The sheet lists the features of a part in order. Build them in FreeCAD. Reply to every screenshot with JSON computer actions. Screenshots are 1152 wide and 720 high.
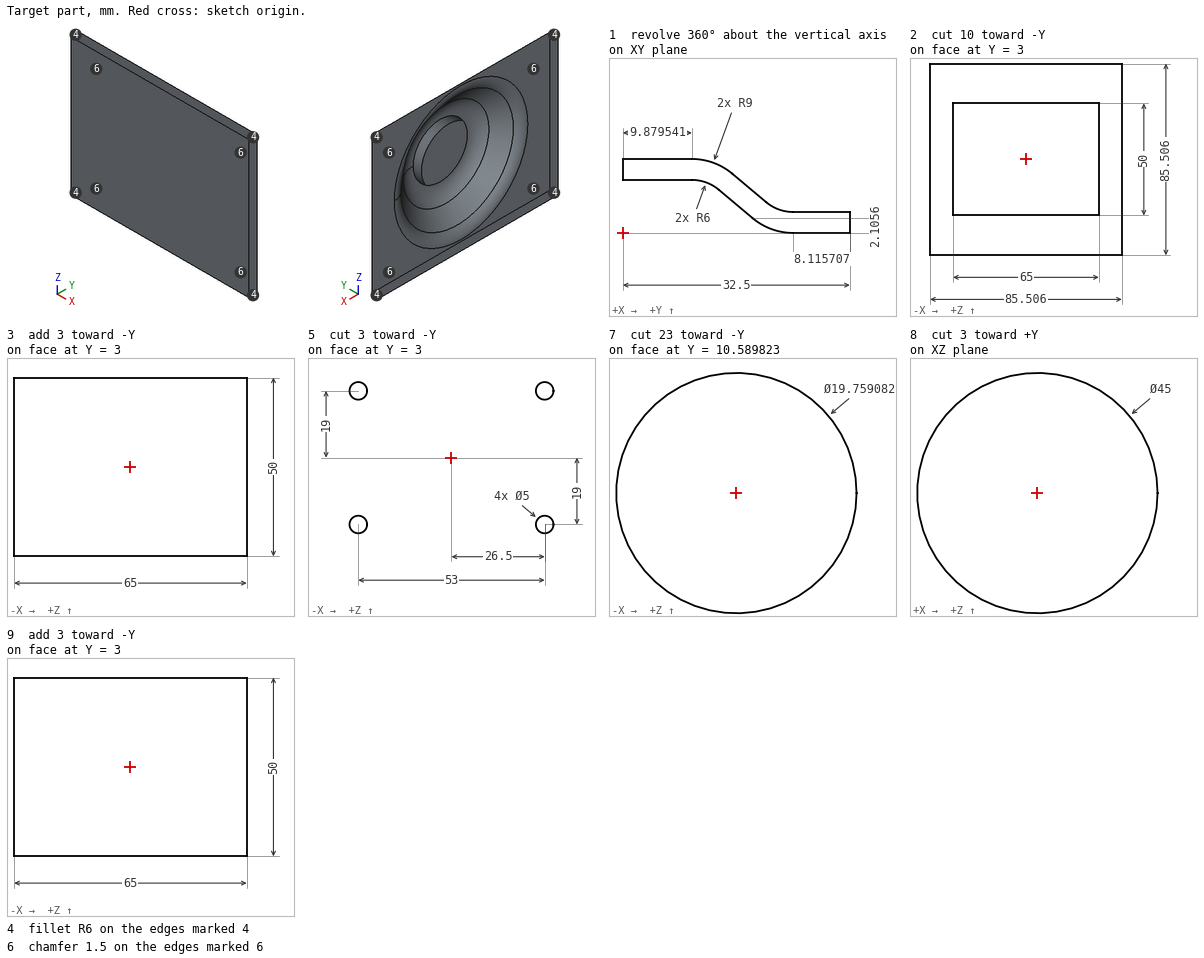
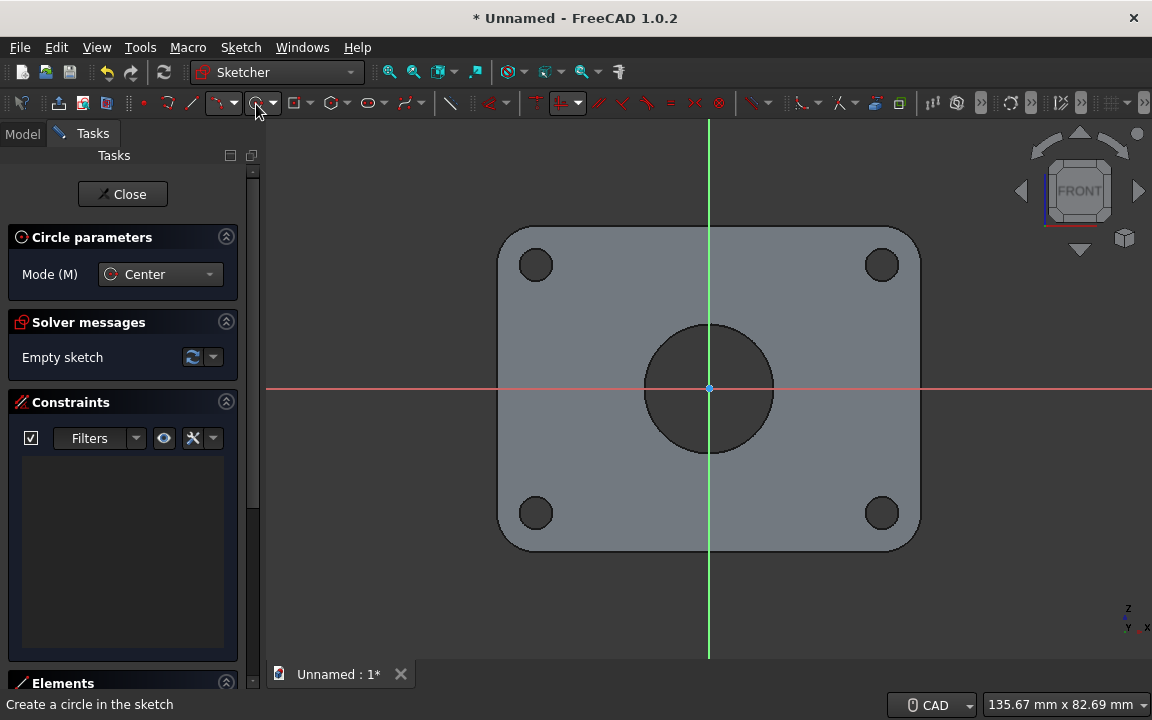
{"action": "left_click", "coordinate": [709, 389]}
{"action": "left_click", "coordinate": [813, 285]}
{"action": "key", "text": "Escape"}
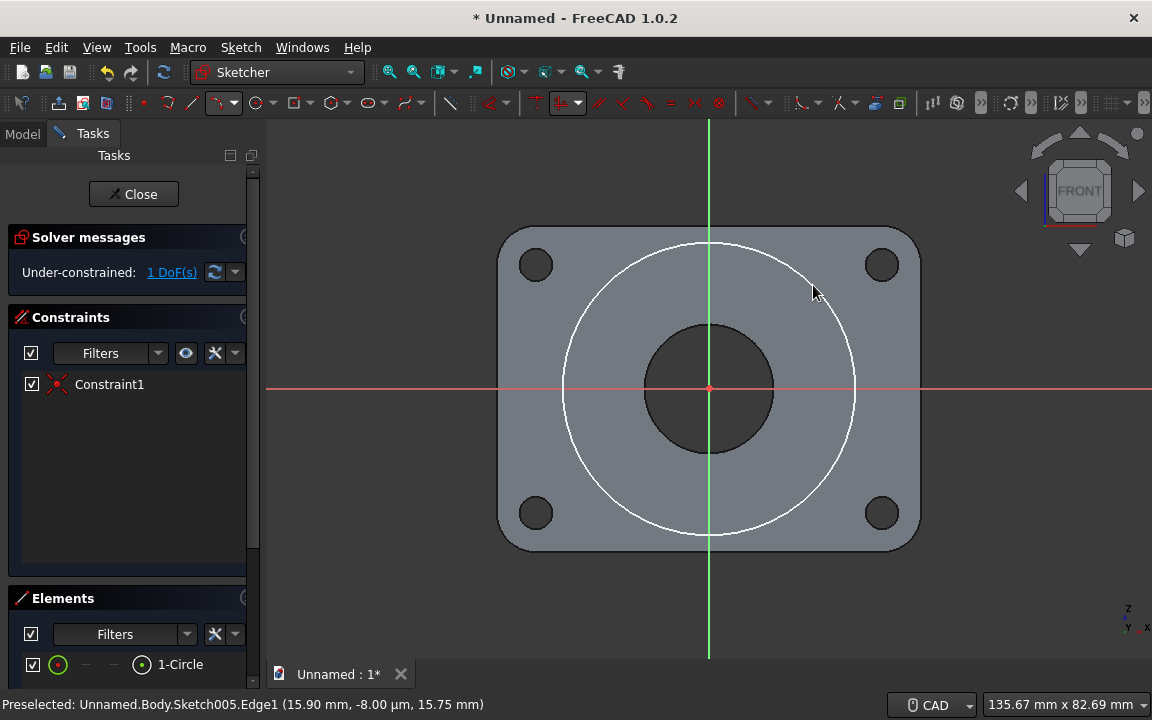
{"action": "left_click", "coordinate": [490, 104]}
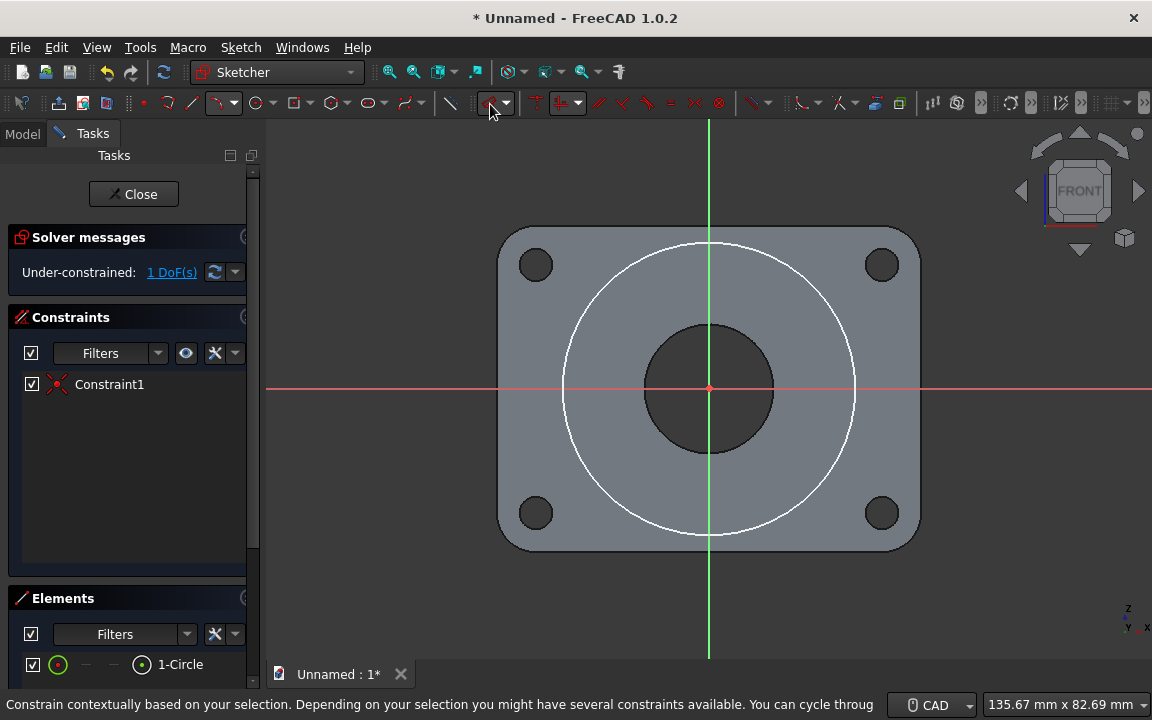
{"action": "left_click", "coordinate": [812, 285]}
{"action": "left_click", "coordinate": [835, 262]}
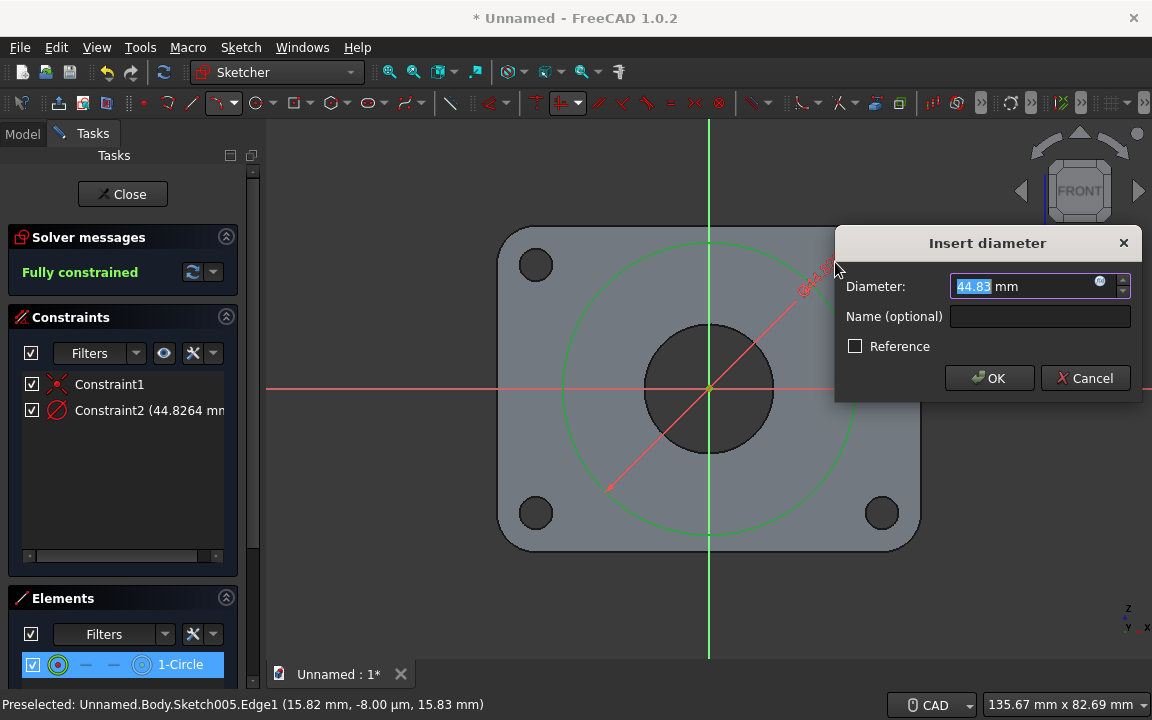
{"action": "type", "text": "45"}
{"action": "key", "text": "Return"}
{"action": "key", "text": "Escape"}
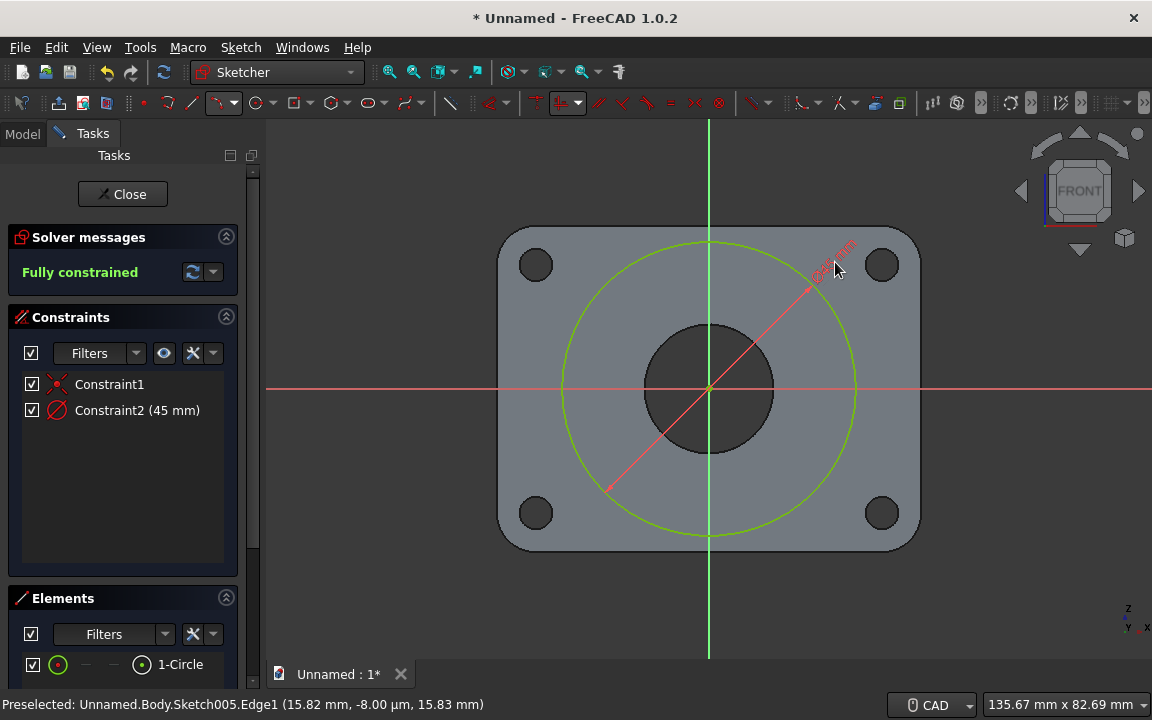
{"action": "left_click", "coordinate": [123, 194]}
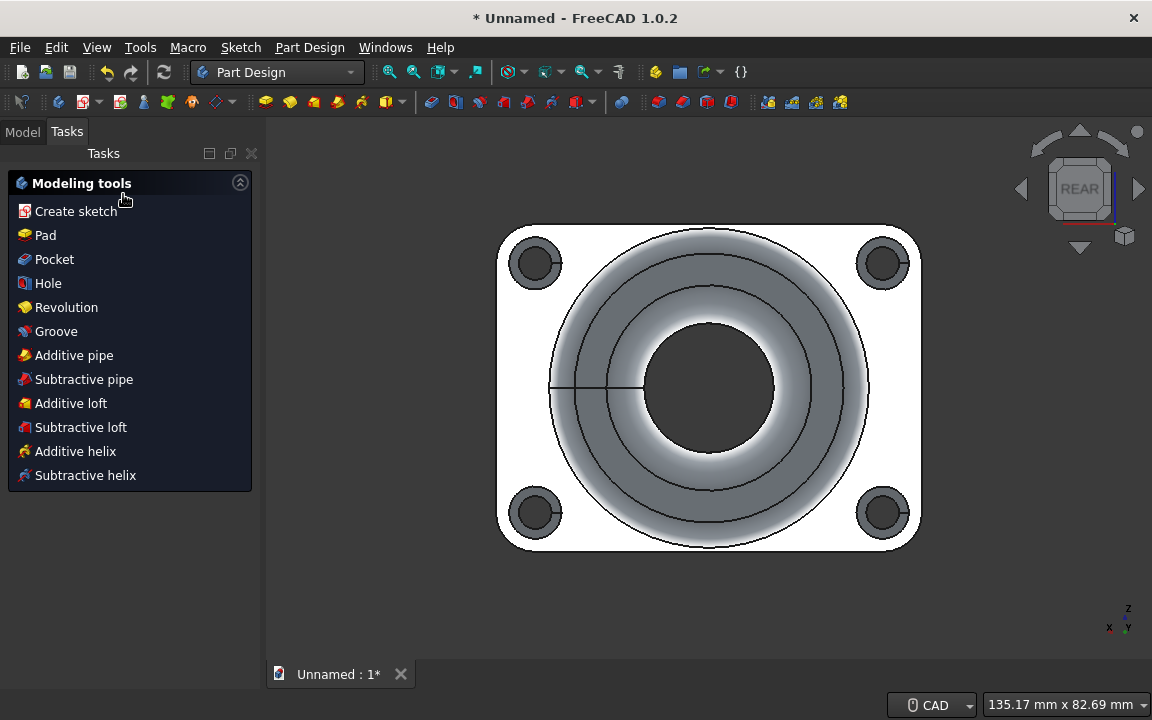
{"action": "left_click", "coordinate": [432, 102]}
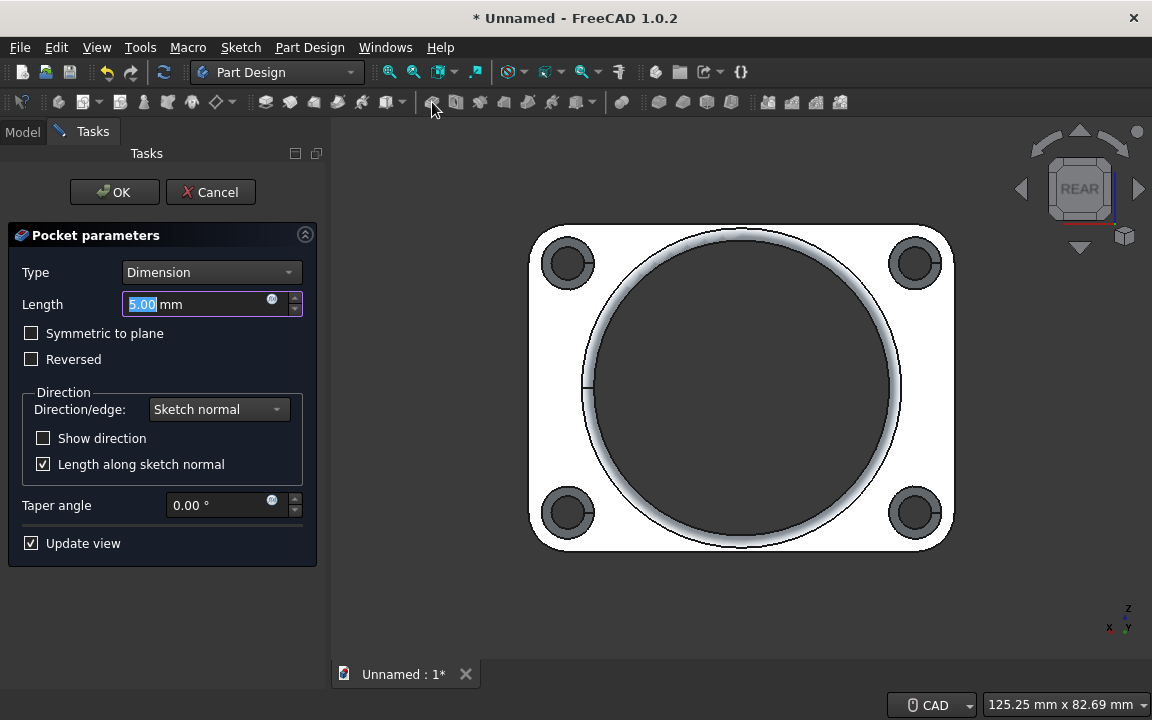
{"action": "type", "text": "3"}
{"action": "key", "text": "Tab"}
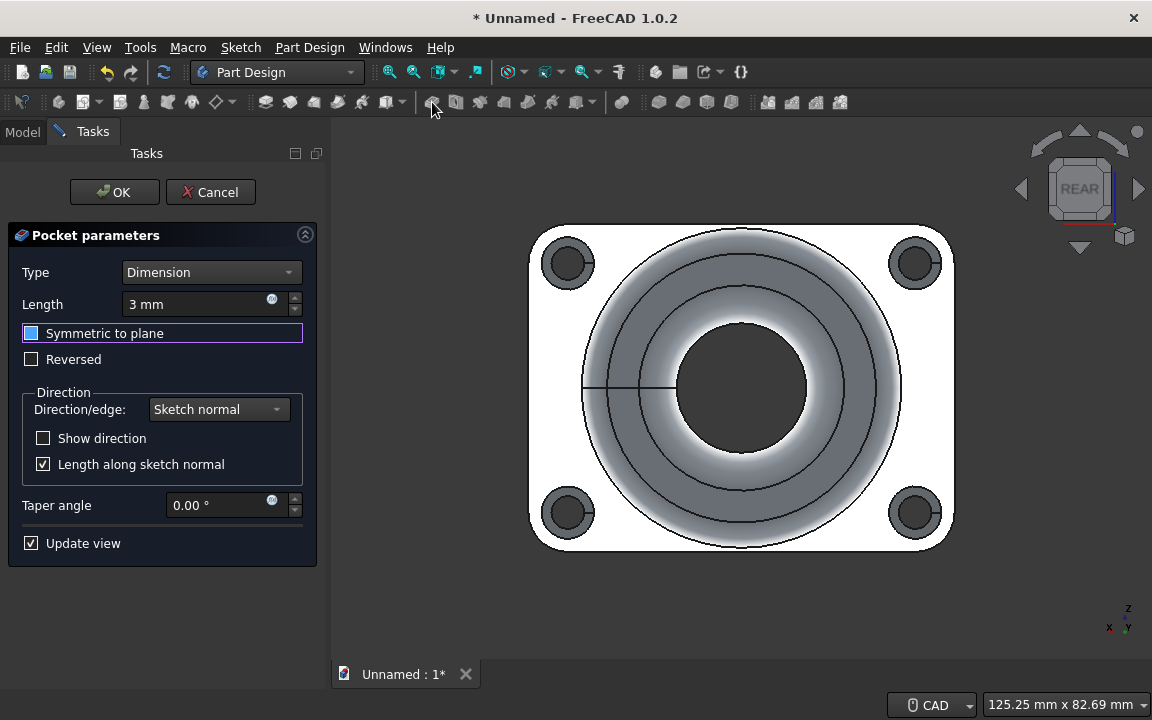
{"action": "left_click", "coordinate": [115, 192]}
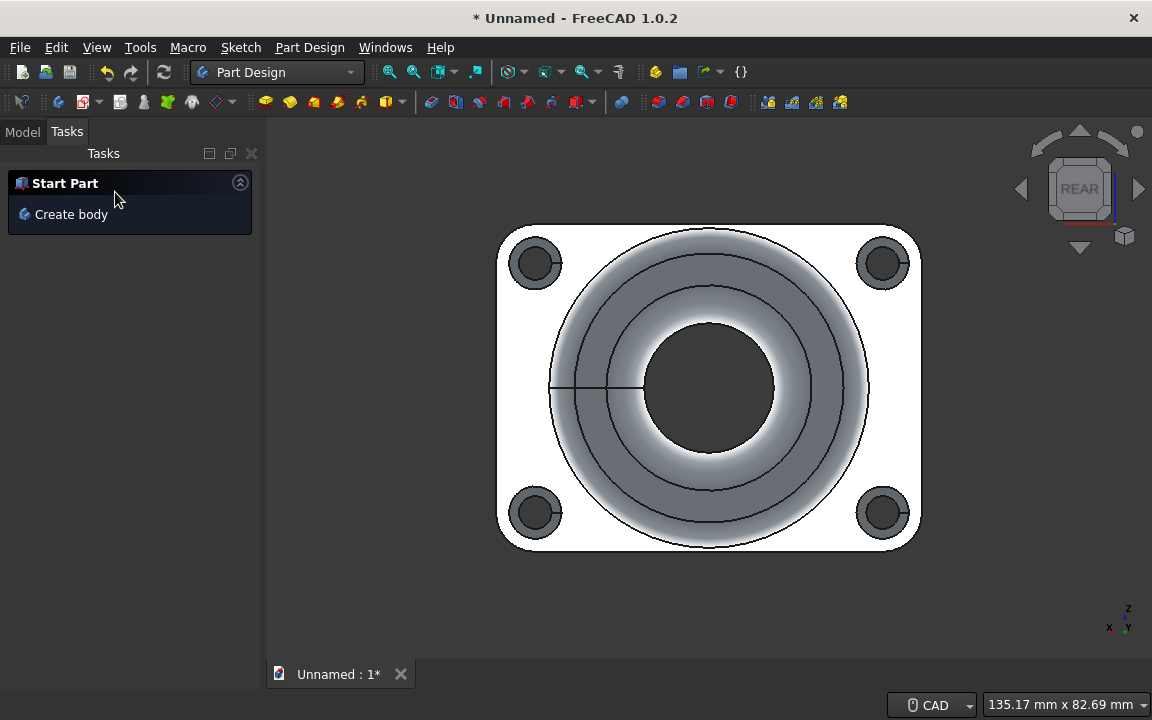
{"action": "left_click", "coordinate": [892, 434]}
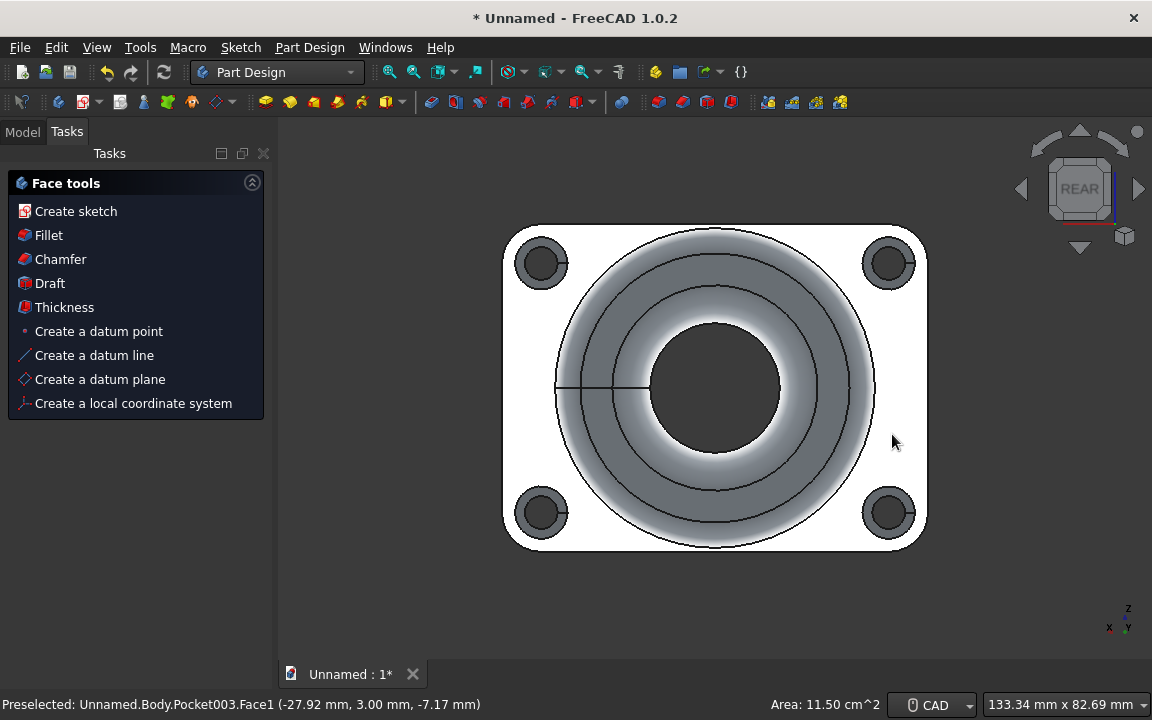
{"action": "left_click", "coordinate": [84, 102]}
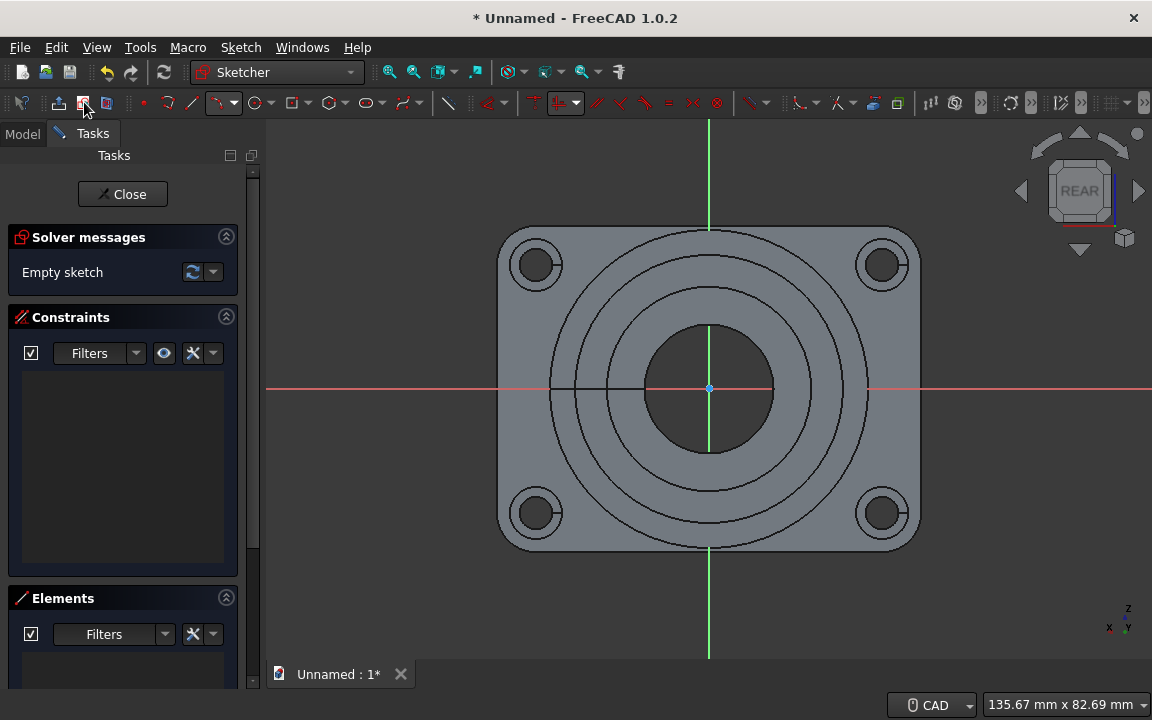
{"action": "left_click", "coordinate": [108, 104]}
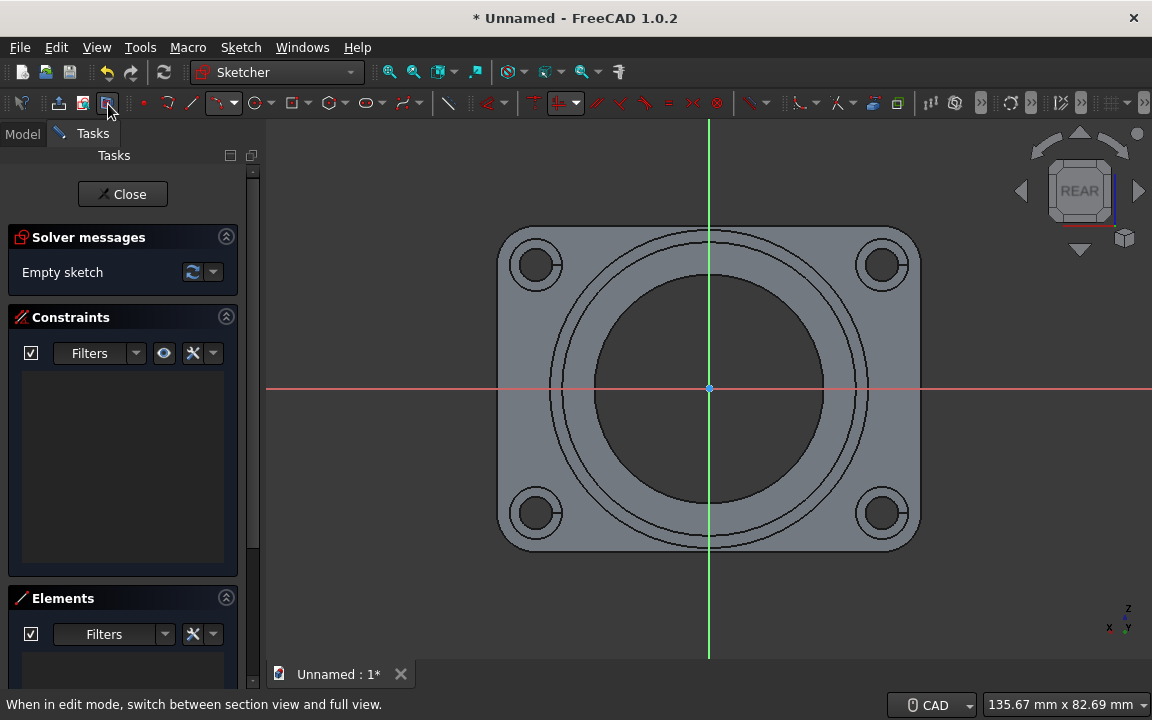
{"action": "left_click", "coordinate": [292, 104]}